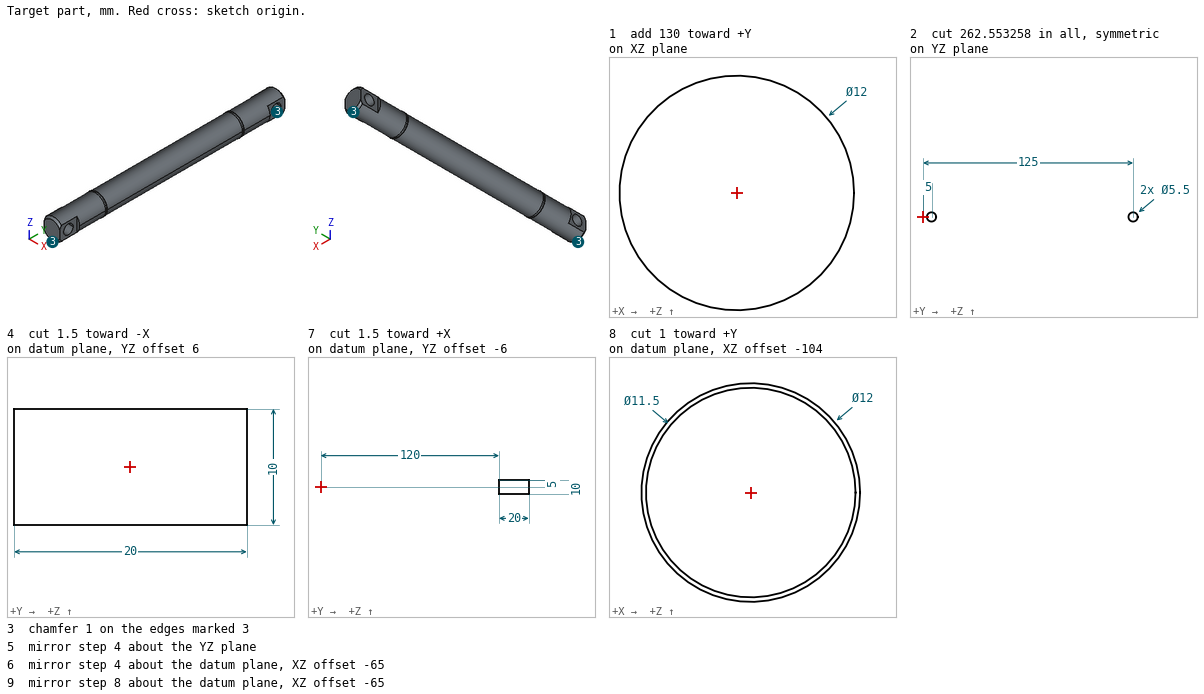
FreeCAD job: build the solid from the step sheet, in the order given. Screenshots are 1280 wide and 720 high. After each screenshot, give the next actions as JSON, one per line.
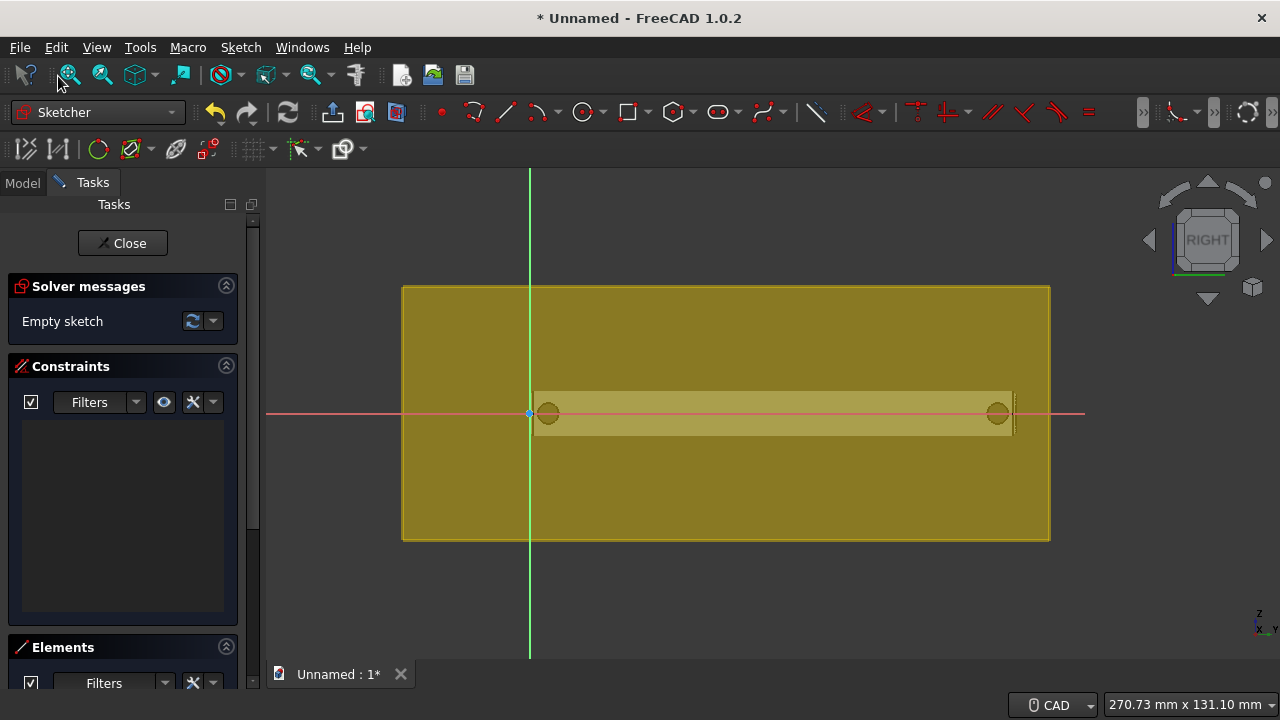
{"action": "scroll", "coordinate": [502, 414], "scroll_direction": "up", "scroll_amount": 10}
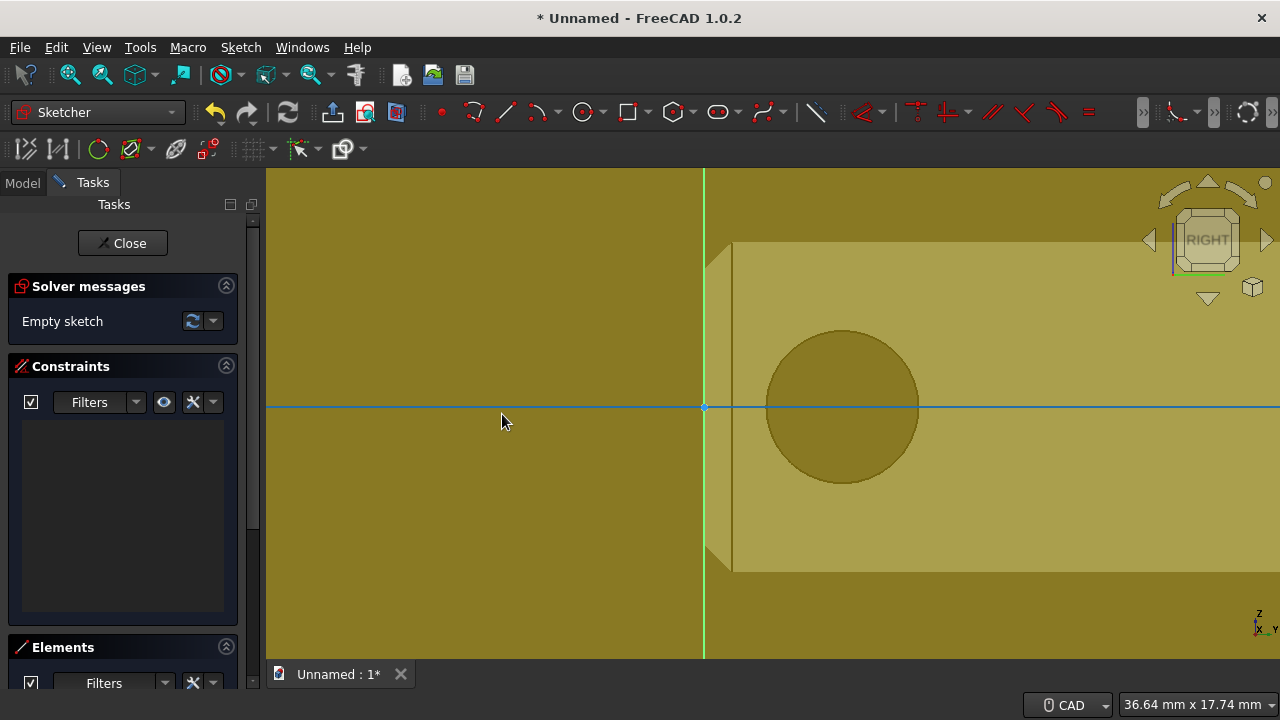
{"action": "key", "text": "g v"}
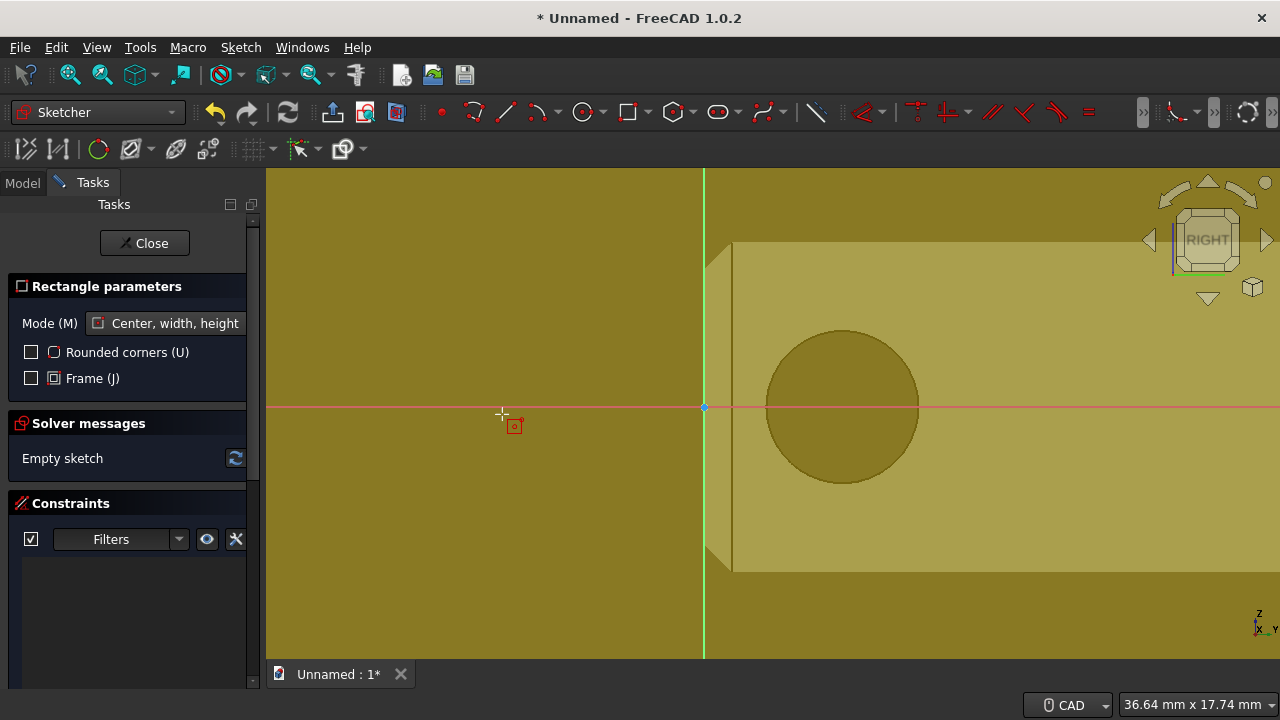
{"action": "left_click", "coordinate": [704, 407]}
{"action": "mouse_move", "coordinate": [981, 269]}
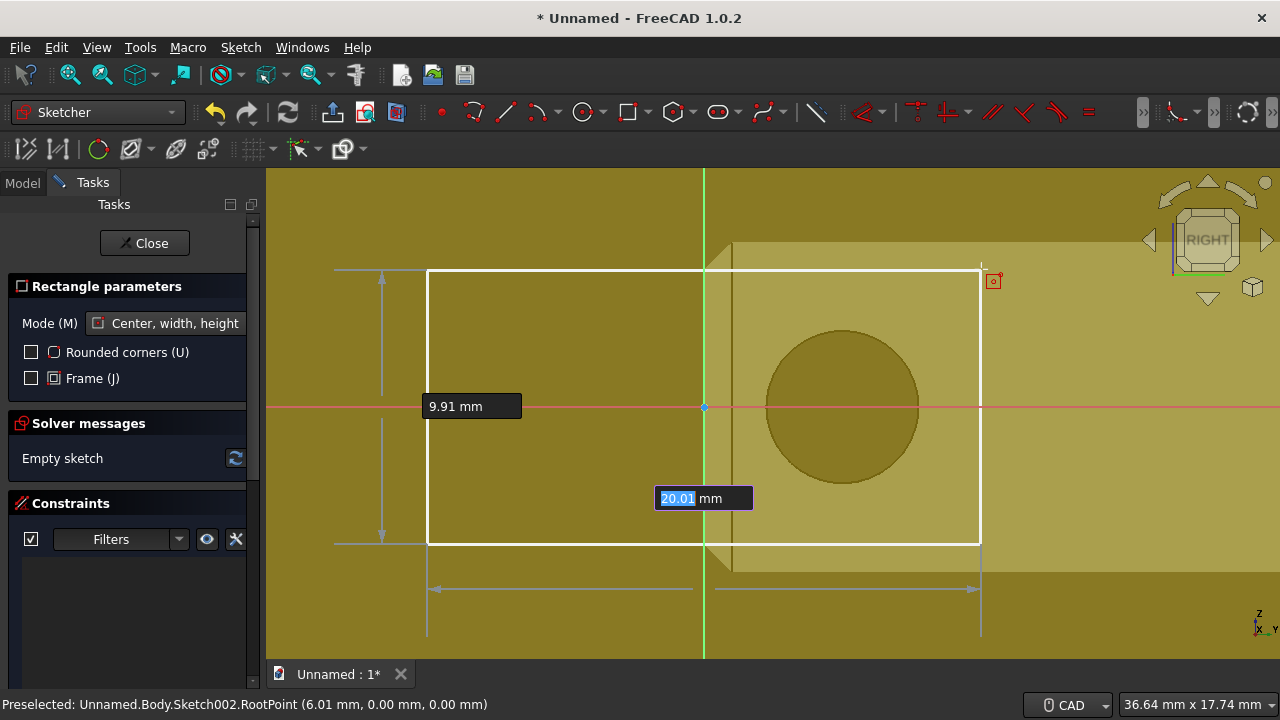
{"action": "type", "text": "20"}
{"action": "key", "text": "Tab"}
{"action": "type", "text": "10"}
{"action": "key", "text": "Return"}
{"action": "key", "text": "Escape"}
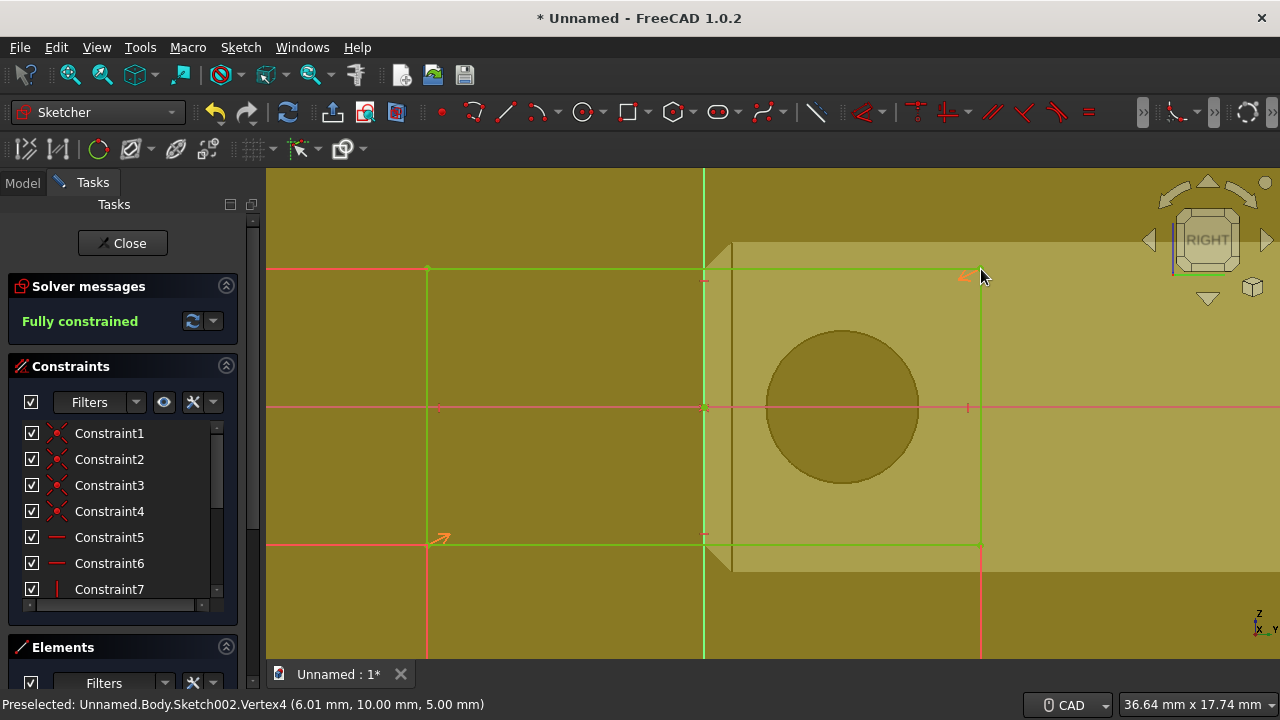
{"action": "left_click", "coordinate": [123, 243]}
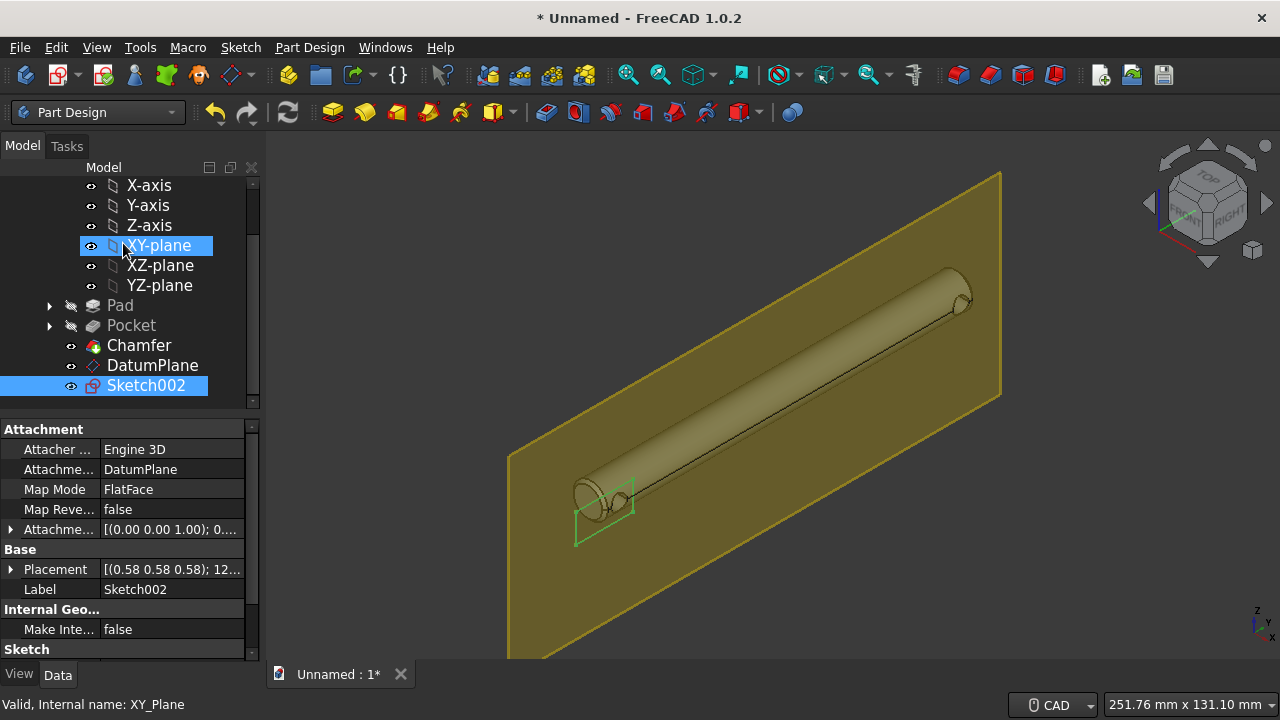
{"action": "left_click", "coordinate": [548, 112]}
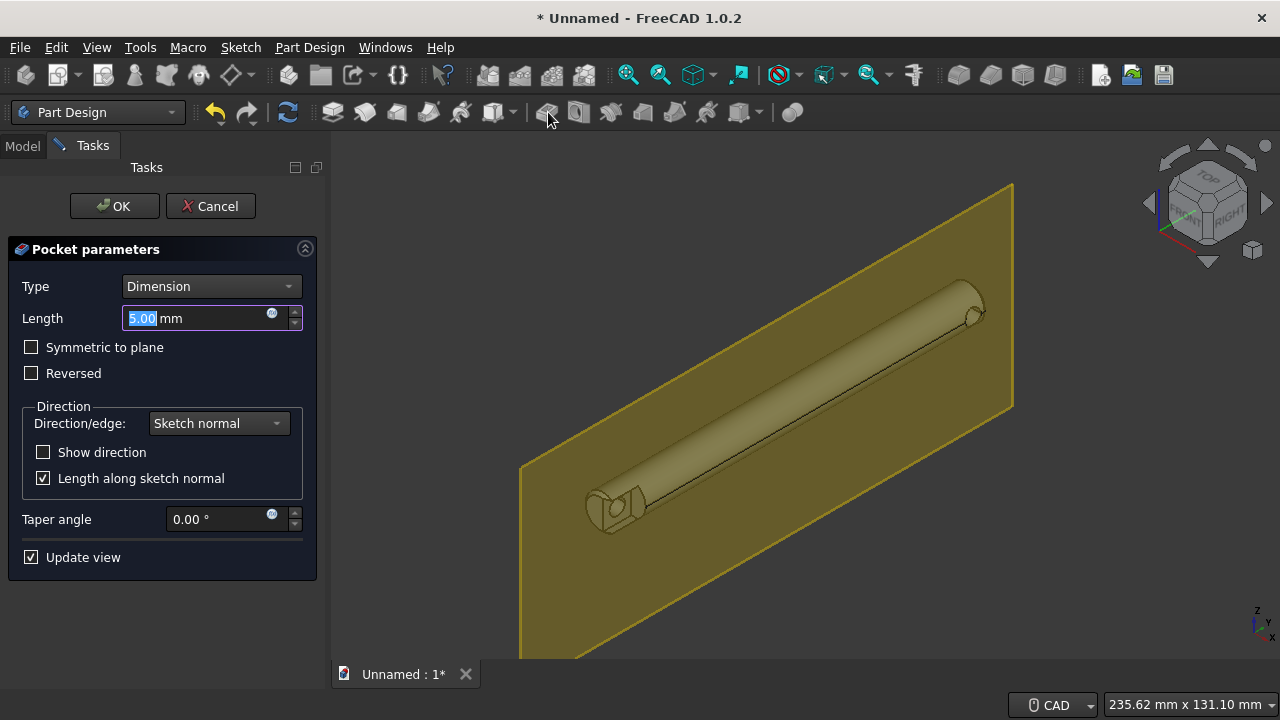
{"action": "type", "text": "1.5"}
{"action": "key", "text": "Tab"}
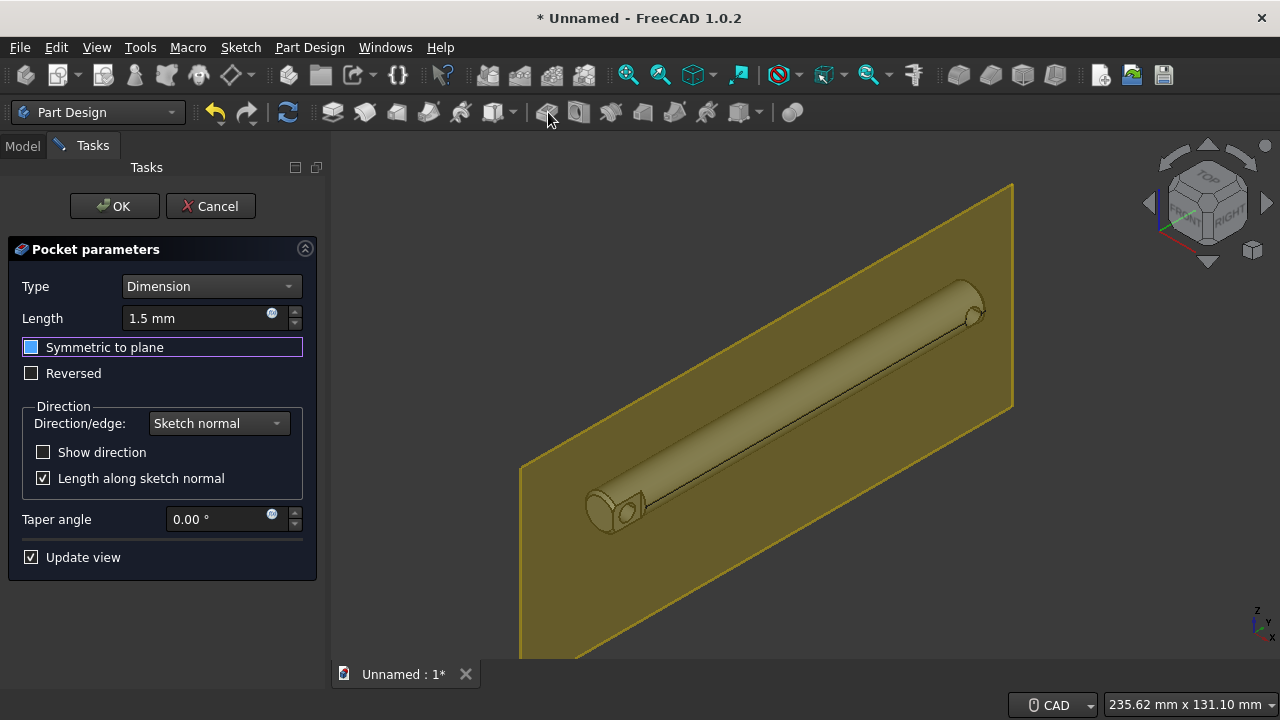
{"action": "left_click", "coordinate": [115, 206]}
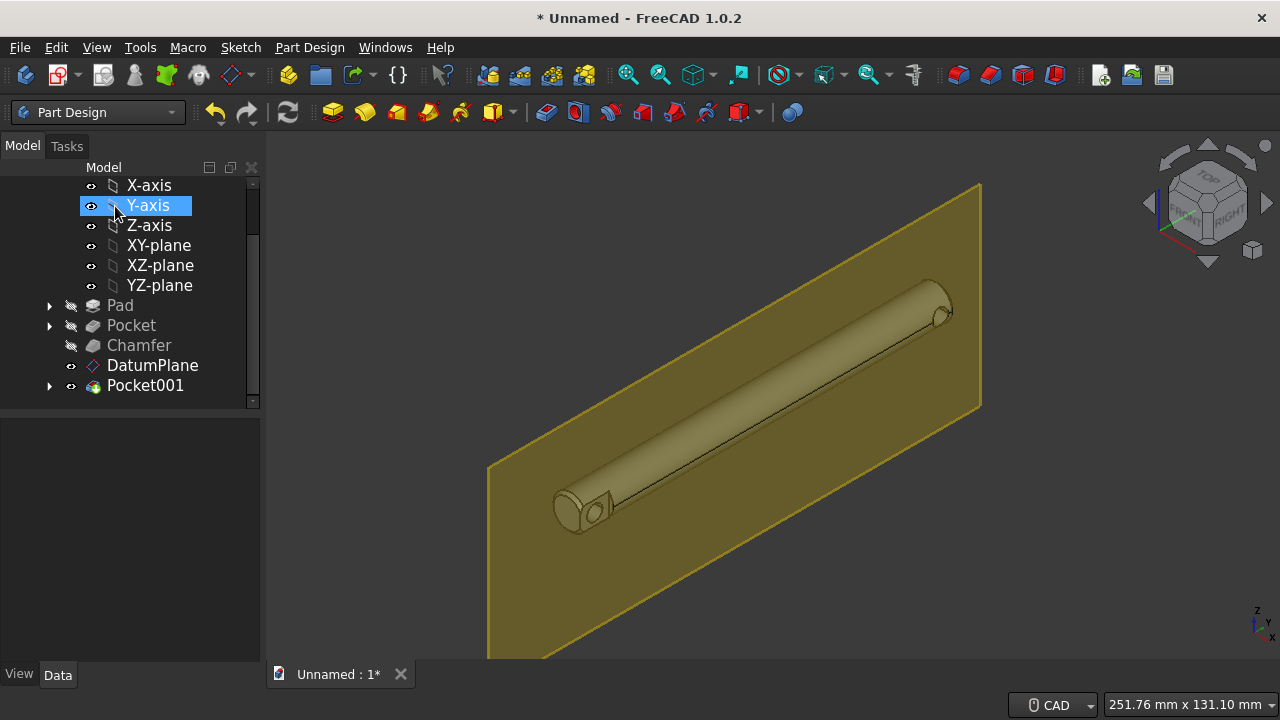
{"action": "left_click", "coordinate": [116, 366]}
{"action": "key", "text": "space"}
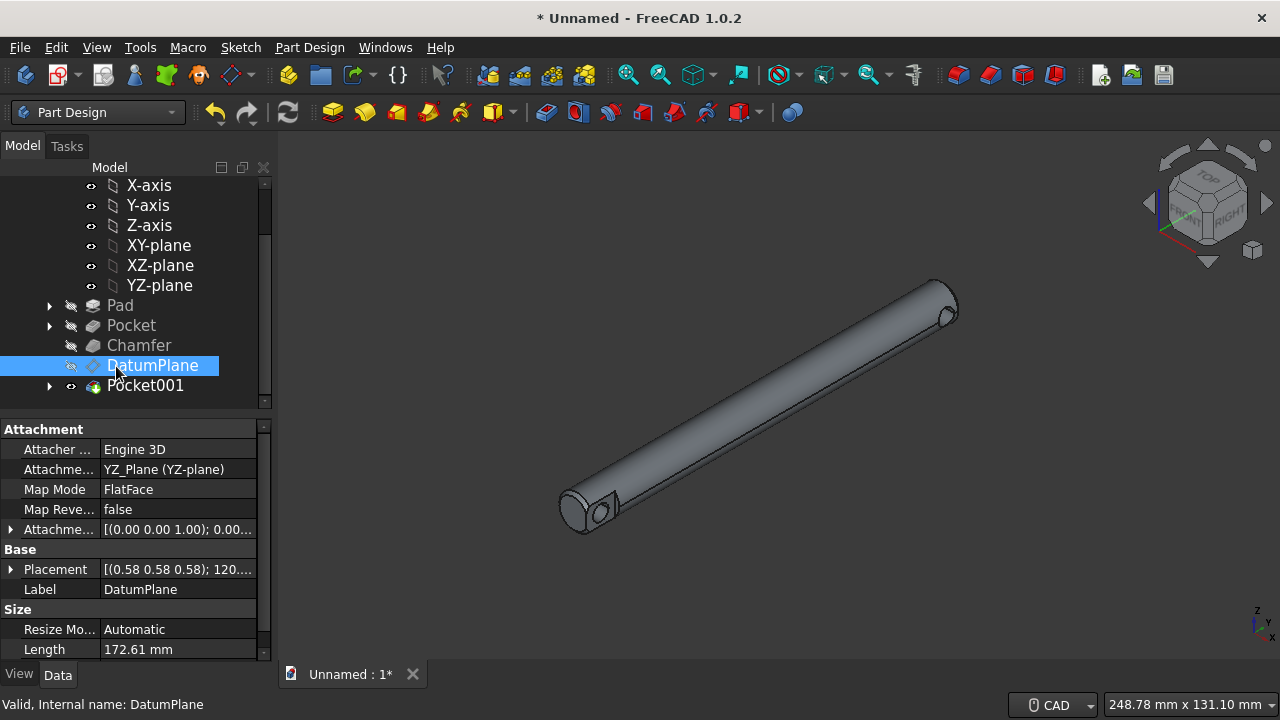
{"action": "left_click", "coordinate": [116, 386]}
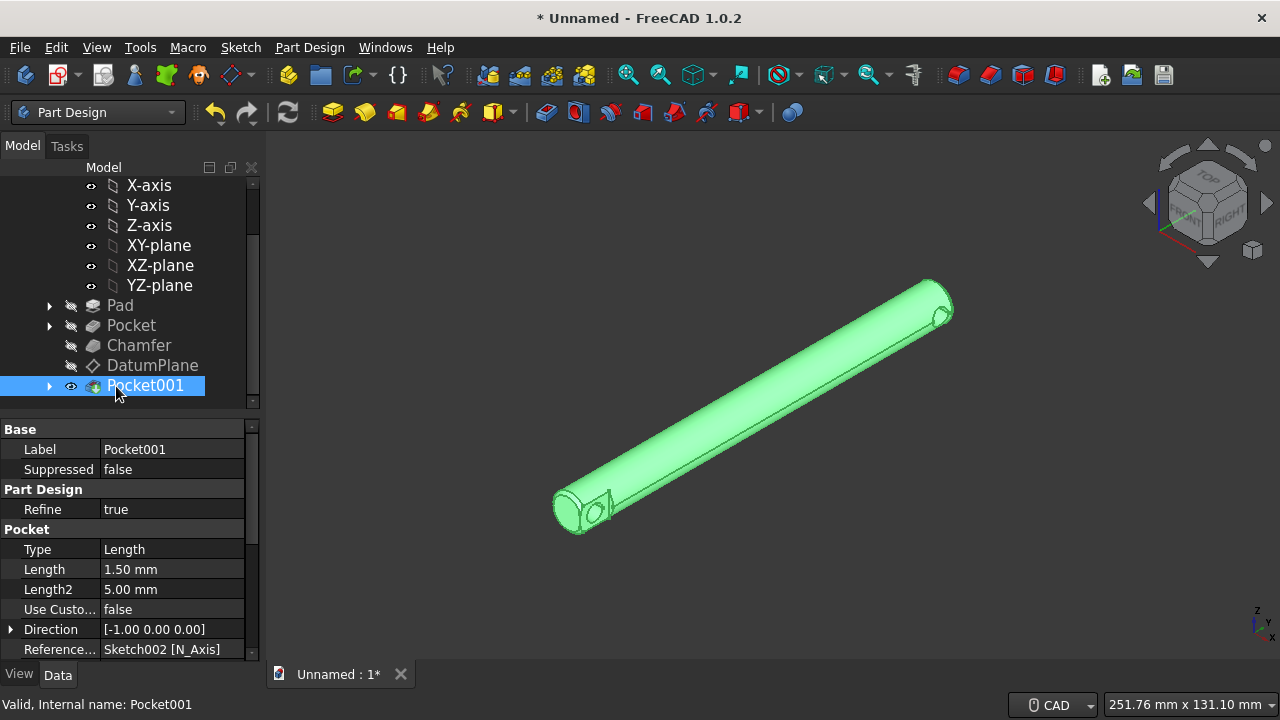
{"action": "left_click", "coordinate": [488, 76]}